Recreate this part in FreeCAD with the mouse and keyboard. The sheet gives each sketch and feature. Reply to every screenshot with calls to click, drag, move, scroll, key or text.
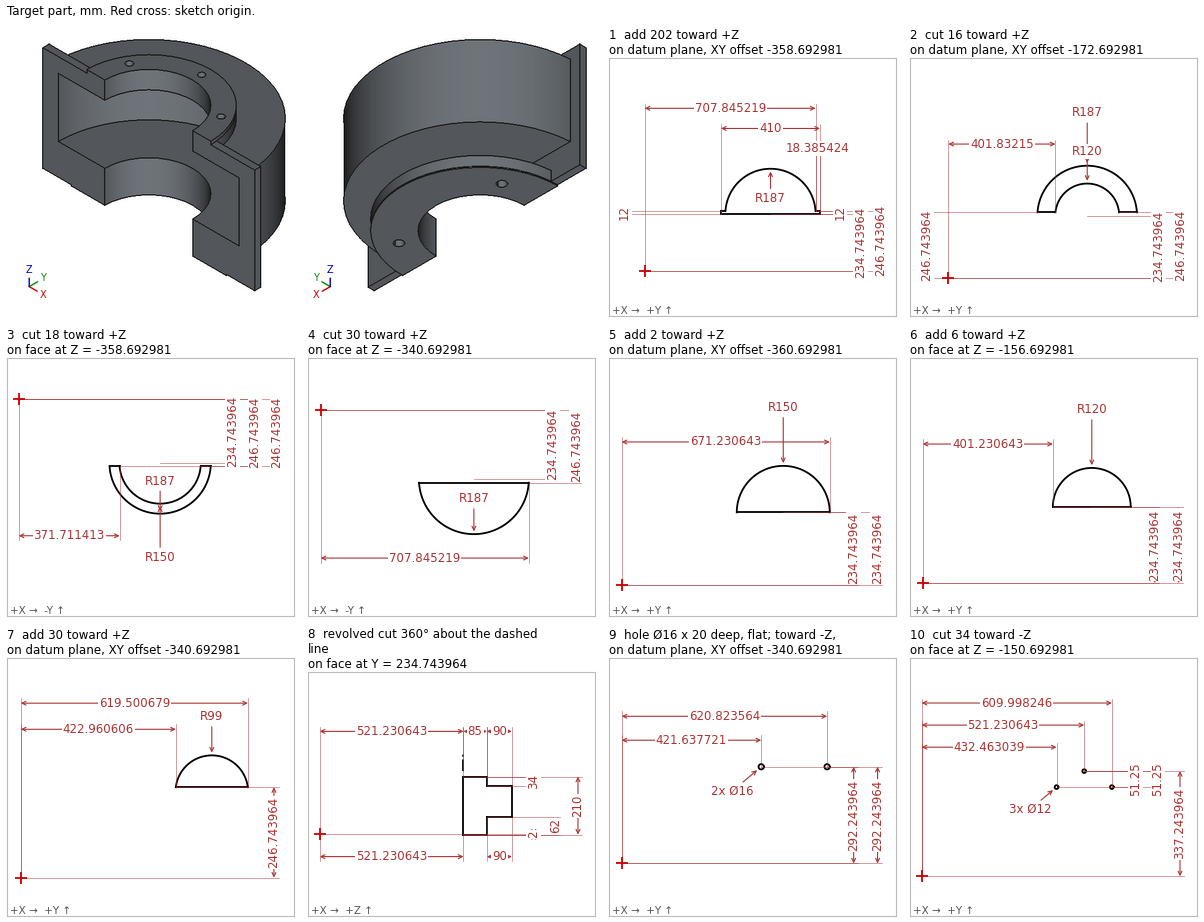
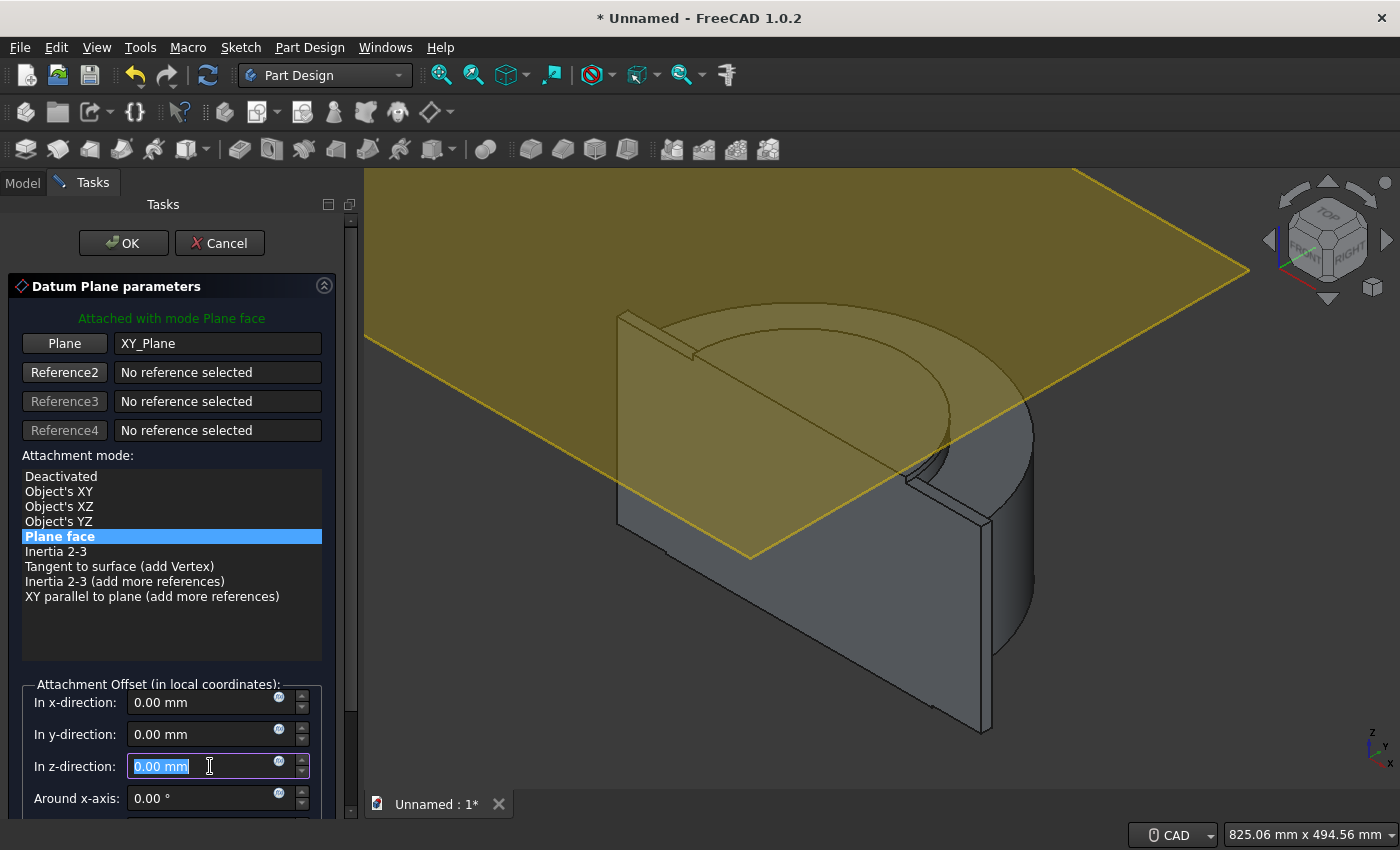
text(-340.692981)
key(Tab)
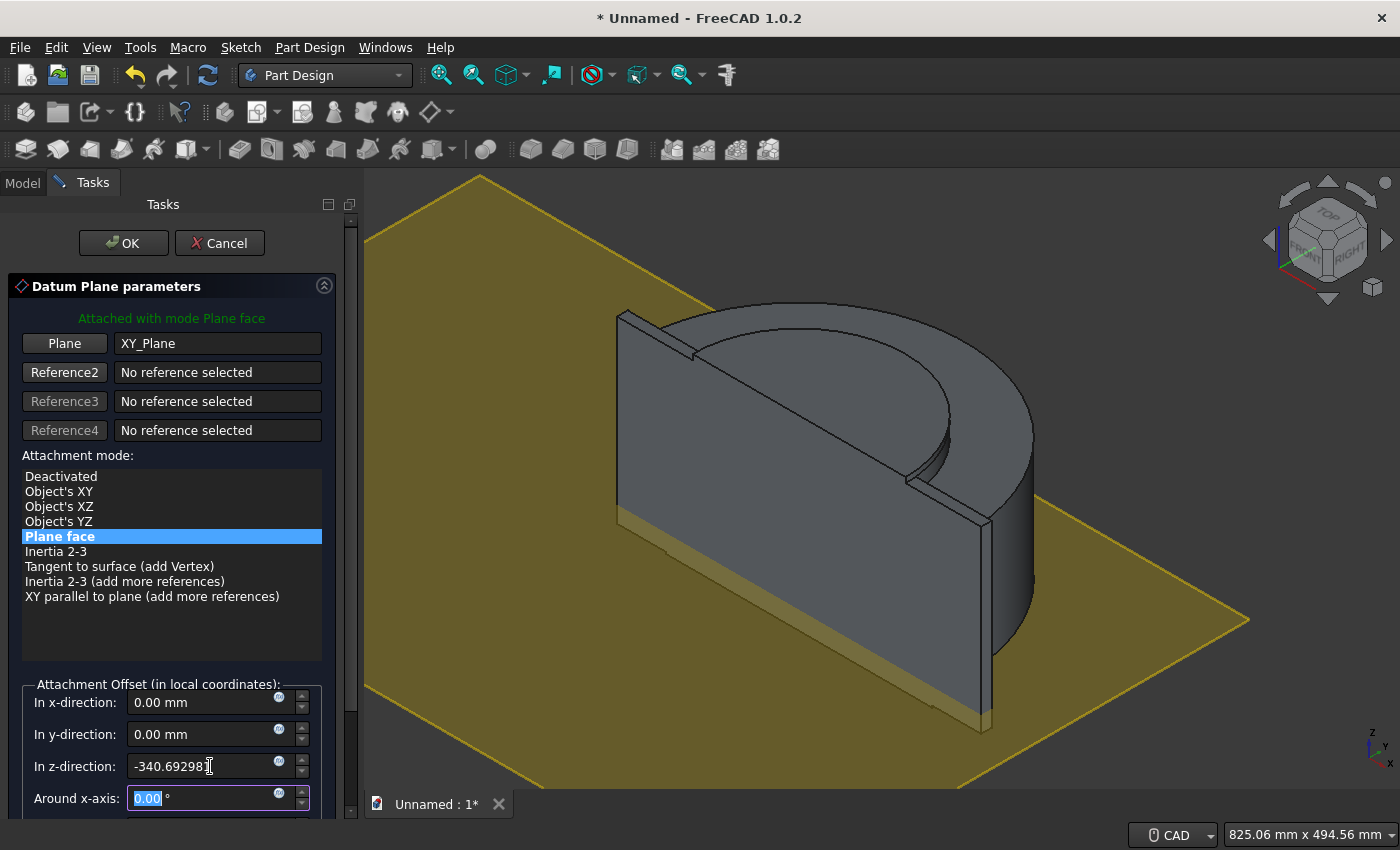
click(124, 243)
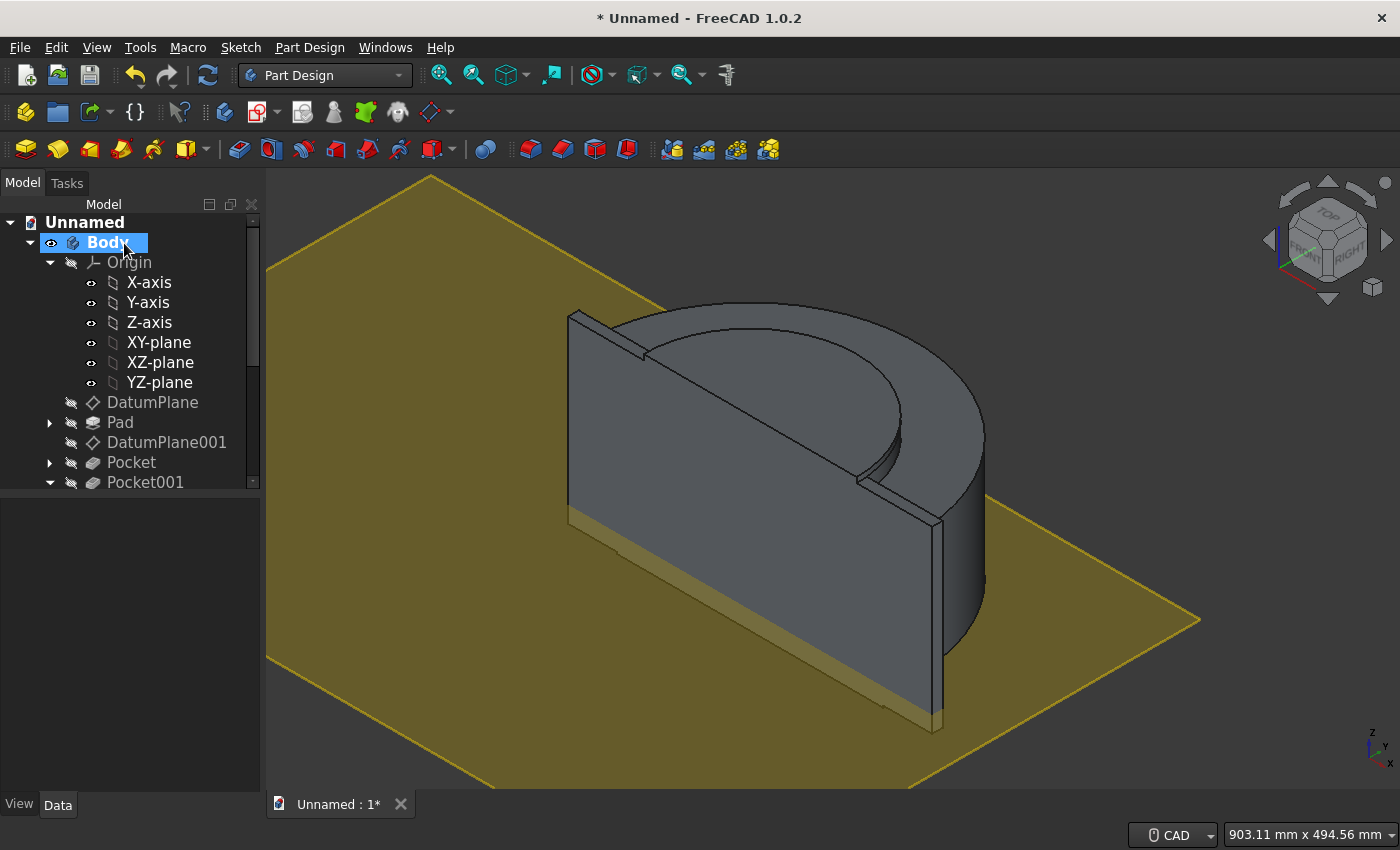
scroll(100, 358, down, 3)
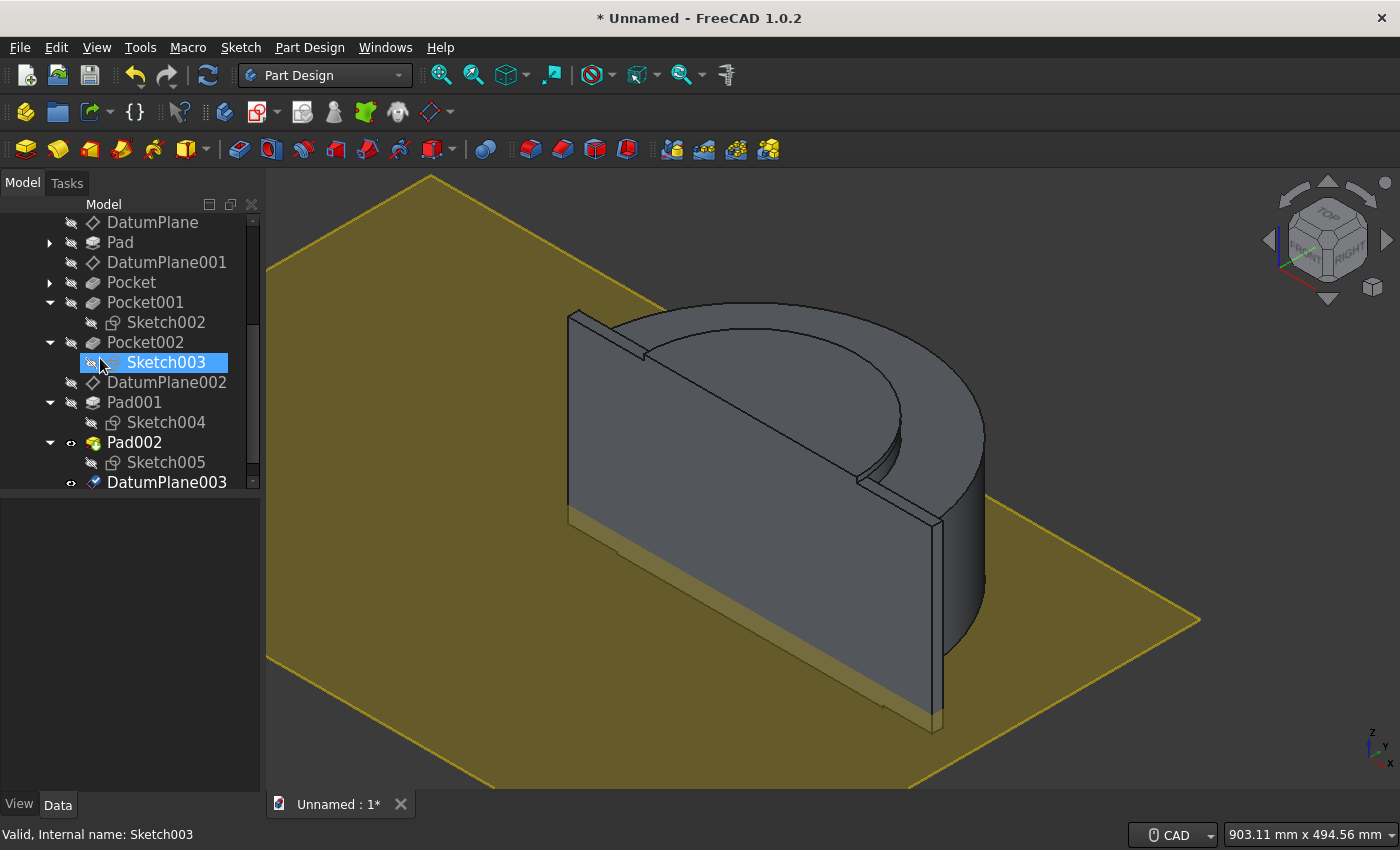
click(116, 483)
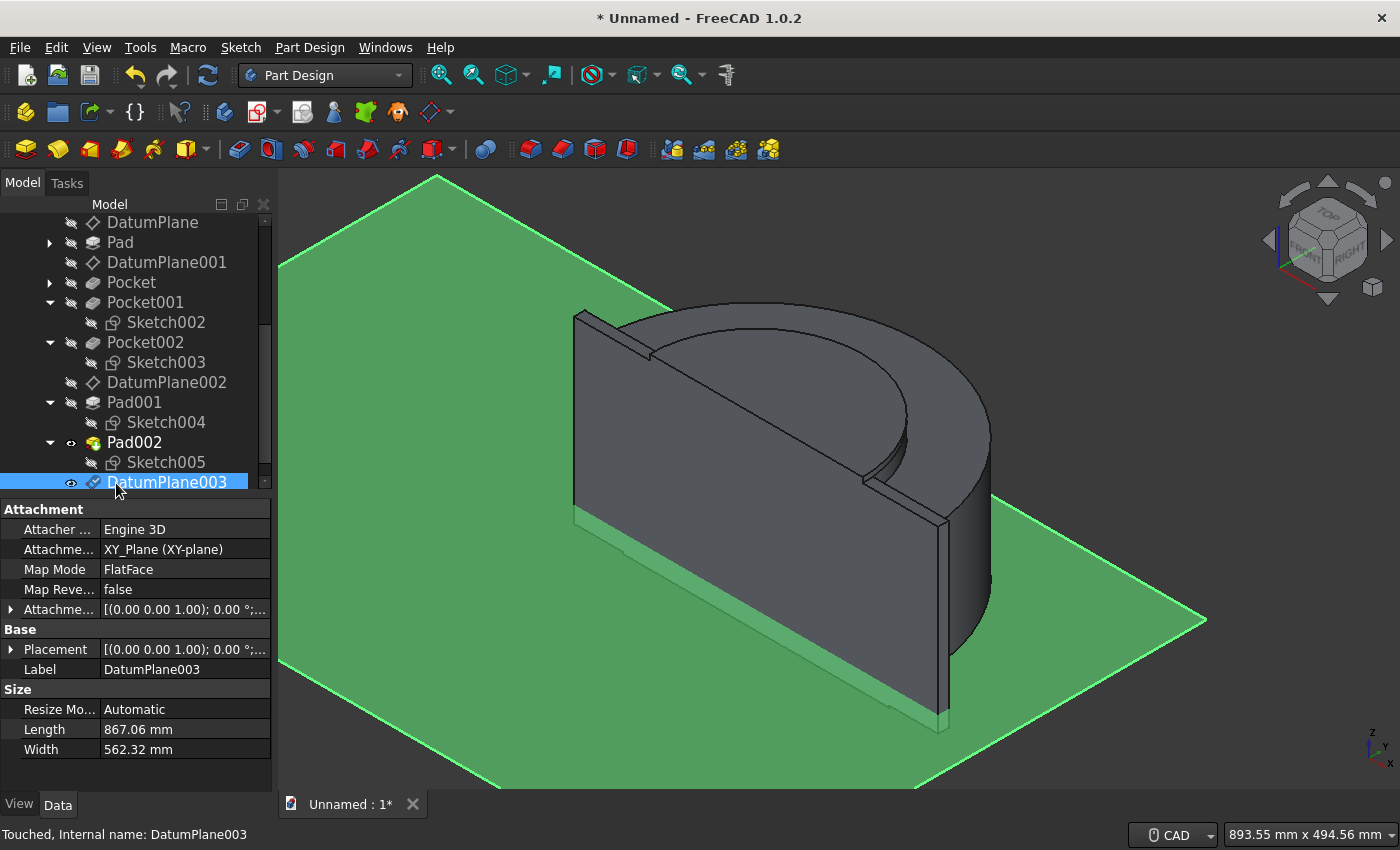
click(258, 112)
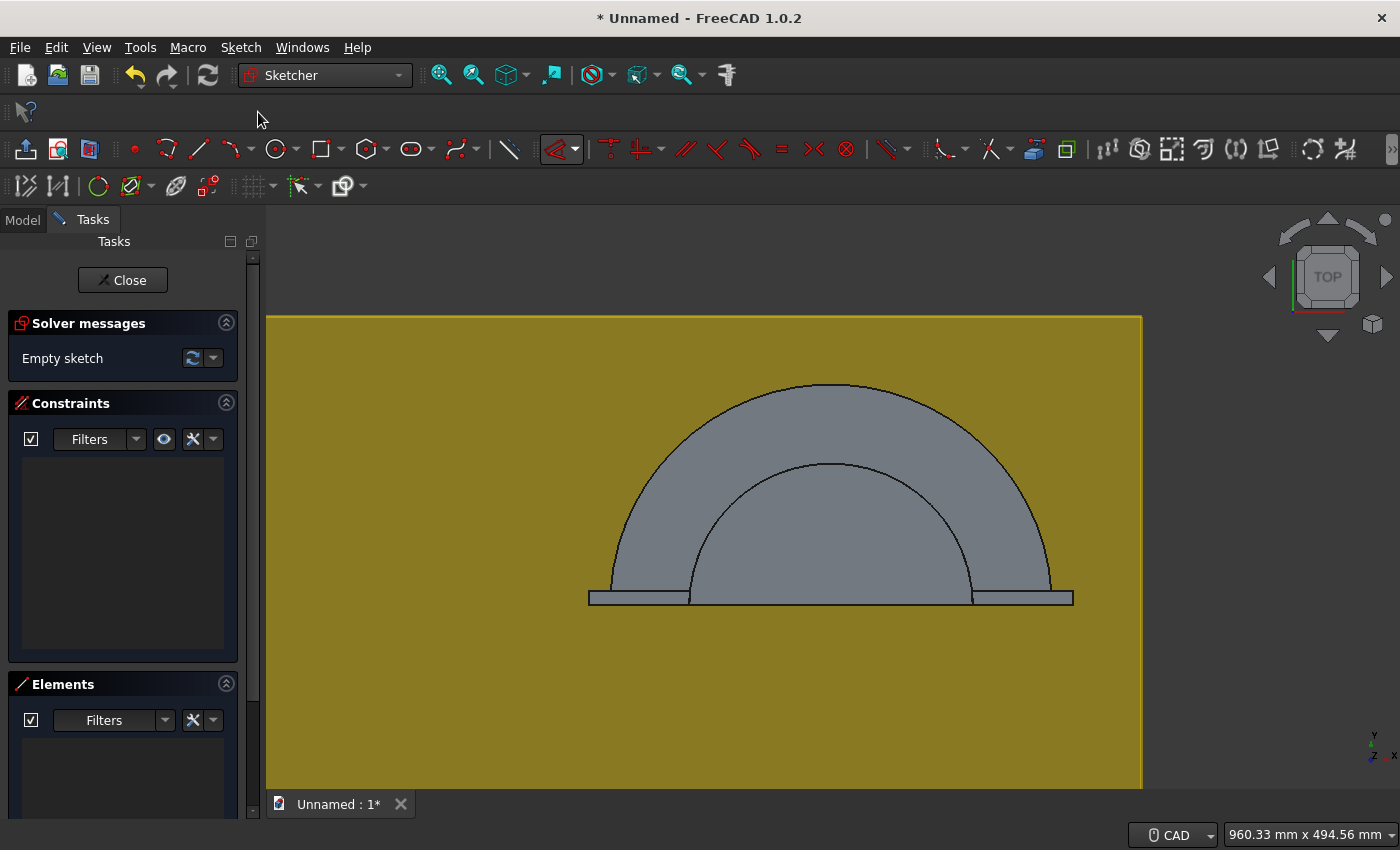
key(q)
key(s)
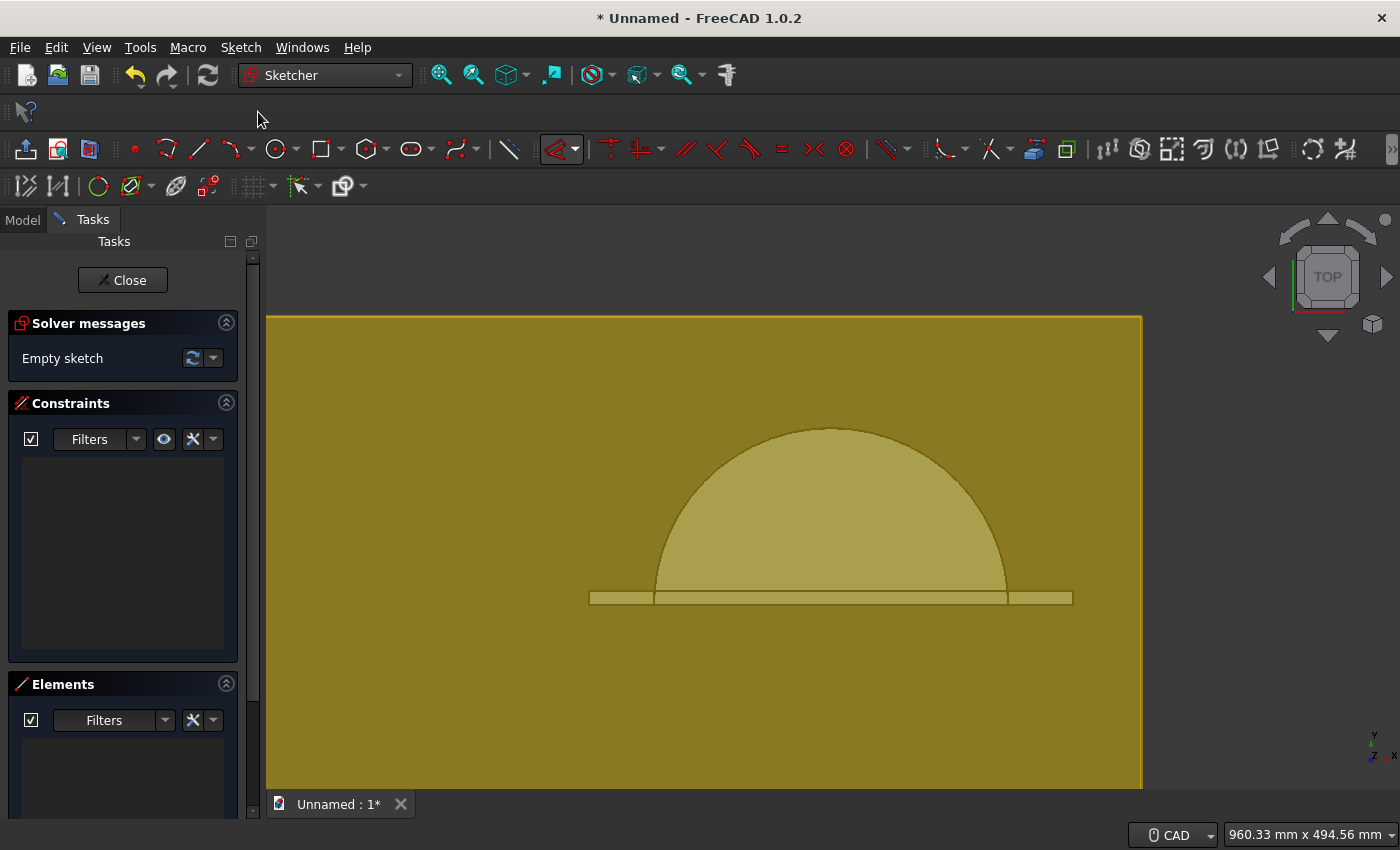
scroll(870, 565, up, 5)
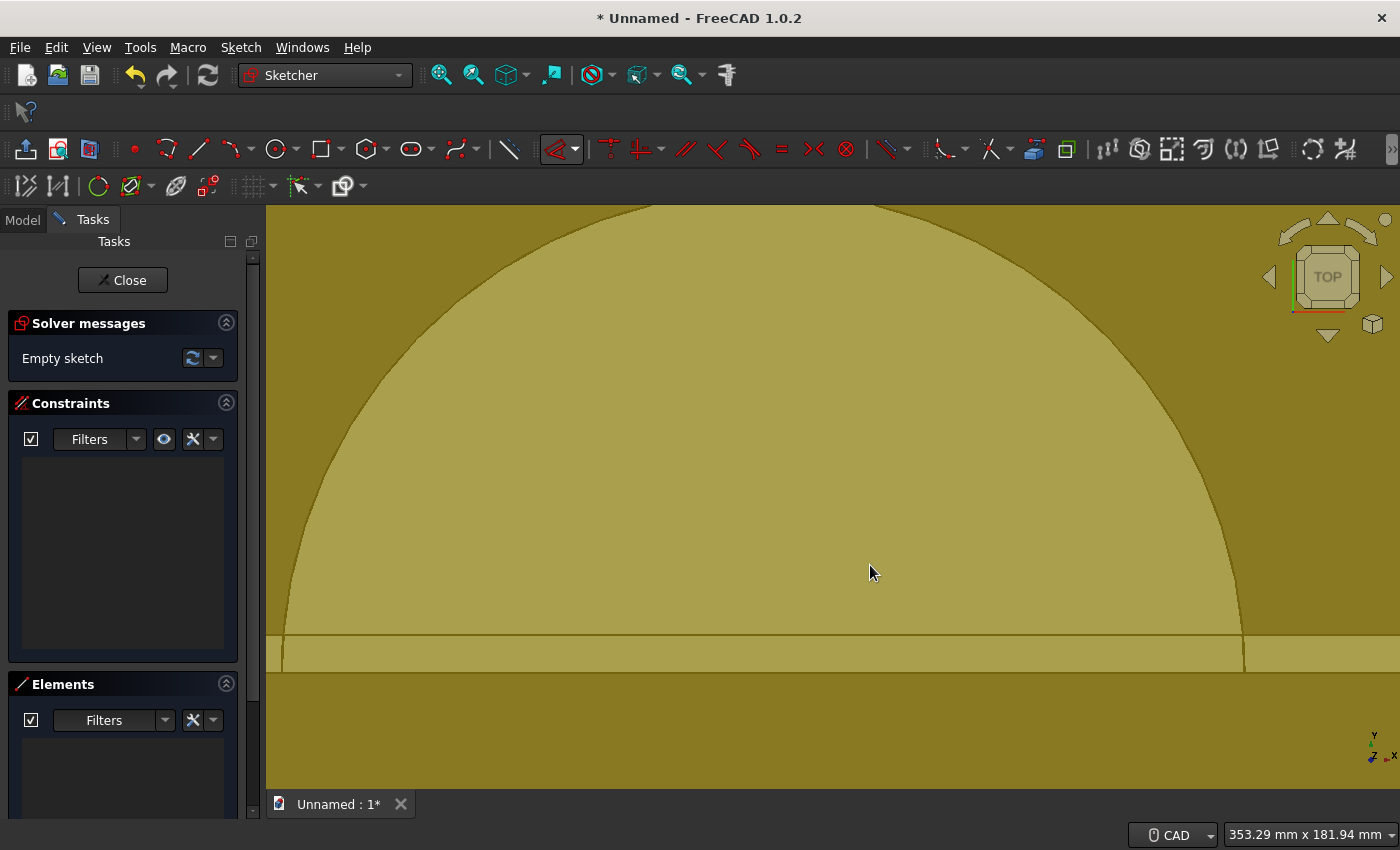
key(g)
key(l)